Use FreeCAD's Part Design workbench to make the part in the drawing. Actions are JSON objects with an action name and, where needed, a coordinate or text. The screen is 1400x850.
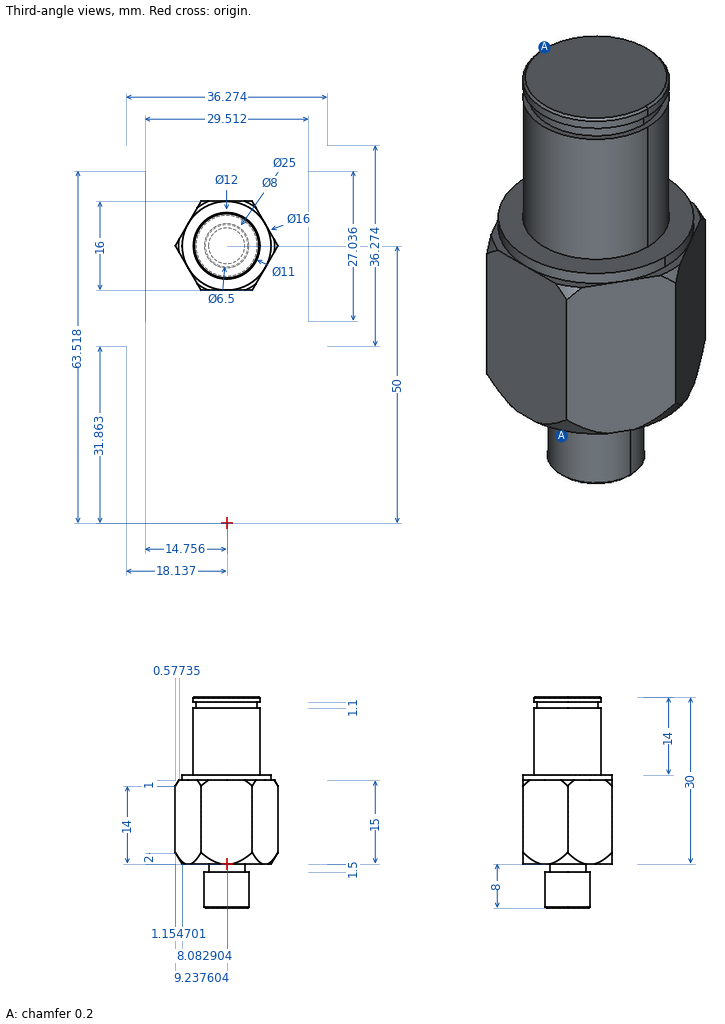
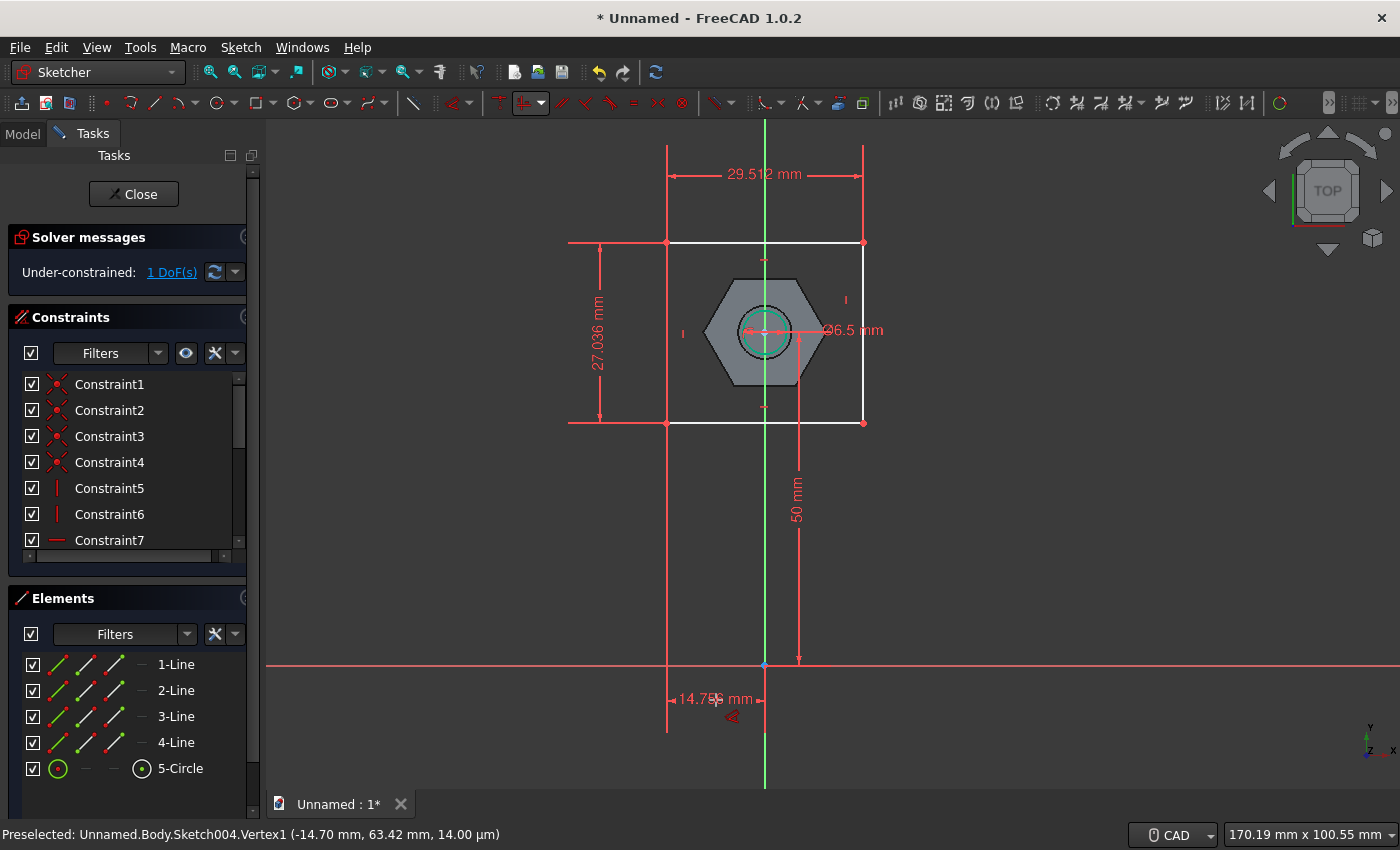
{"action": "left_click", "coordinate": [667, 243]}
{"action": "left_click", "coordinate": [633, 454]}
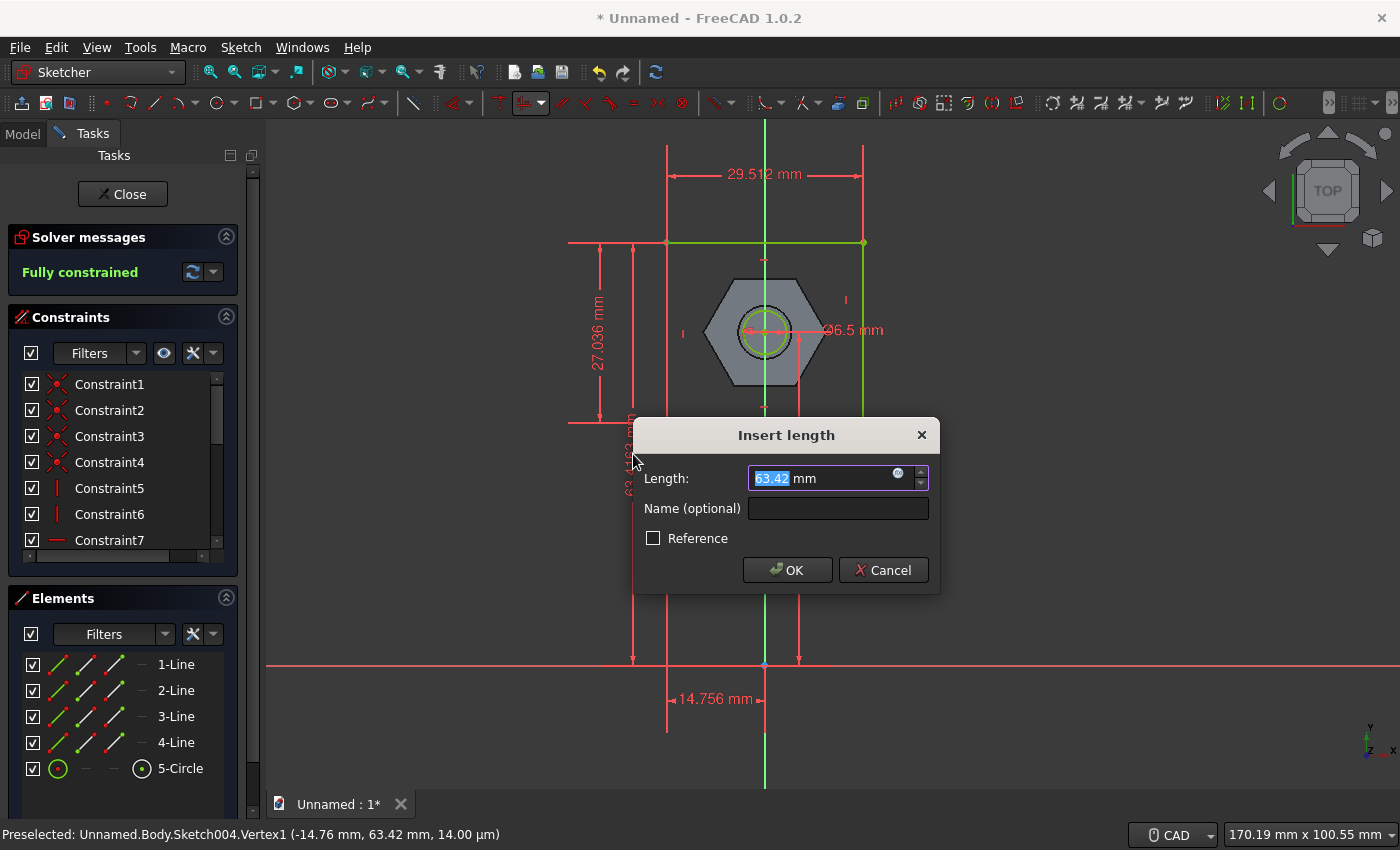
{"action": "type", "text": "63.518"}
{"action": "key", "text": "Return"}
{"action": "key", "text": "Escape"}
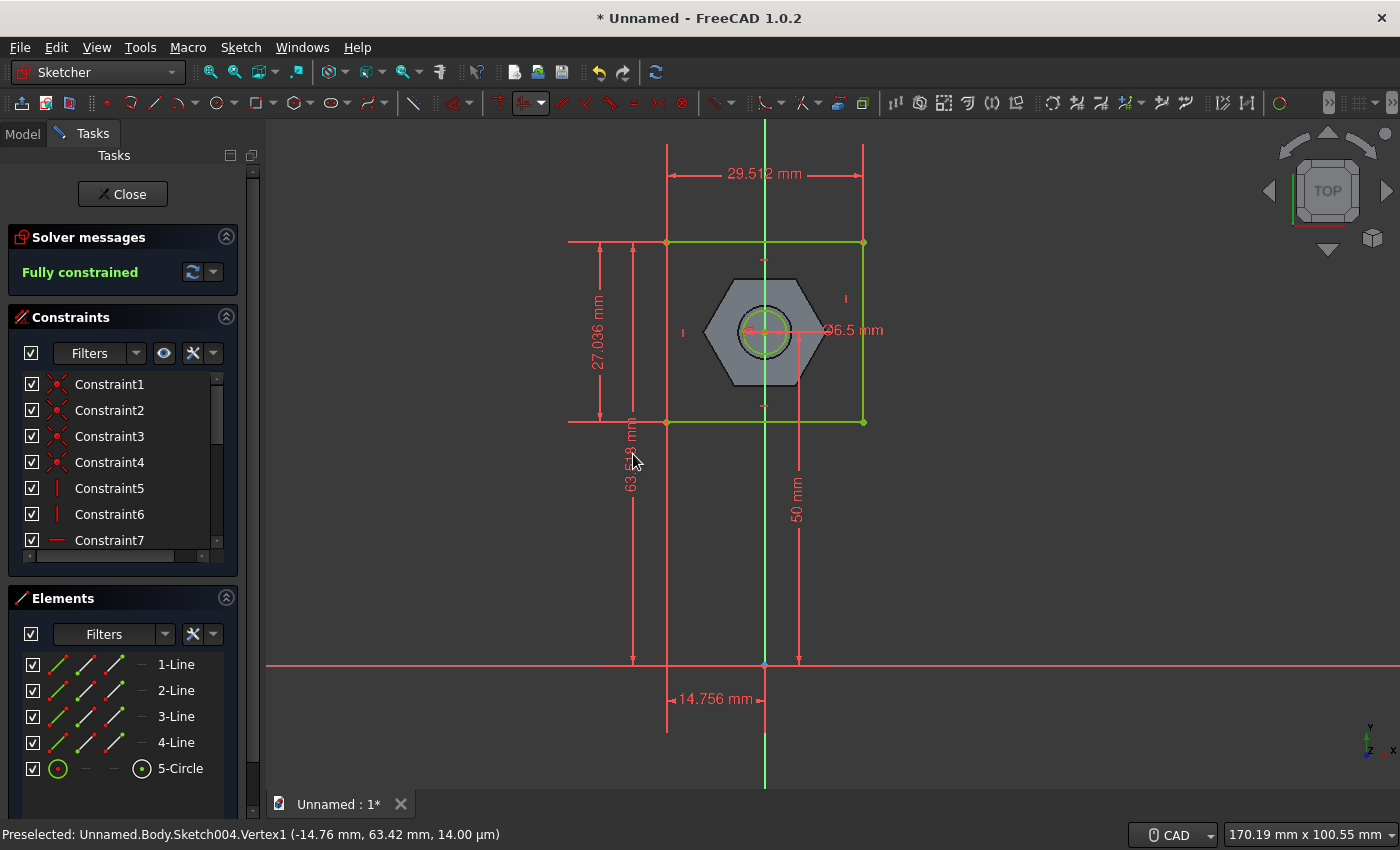
{"action": "left_click", "coordinate": [123, 194]}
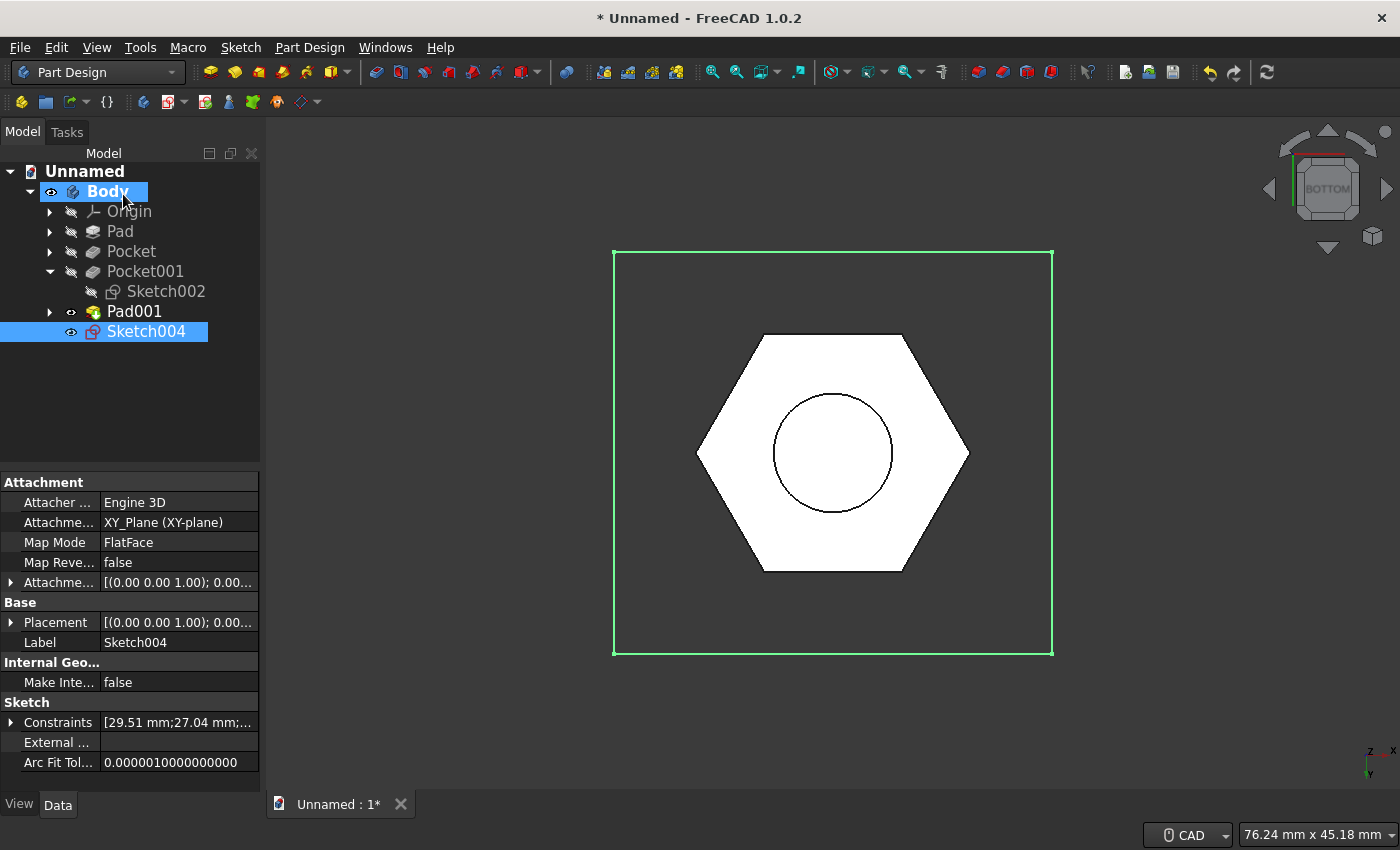
{"action": "left_click", "coordinate": [378, 72]}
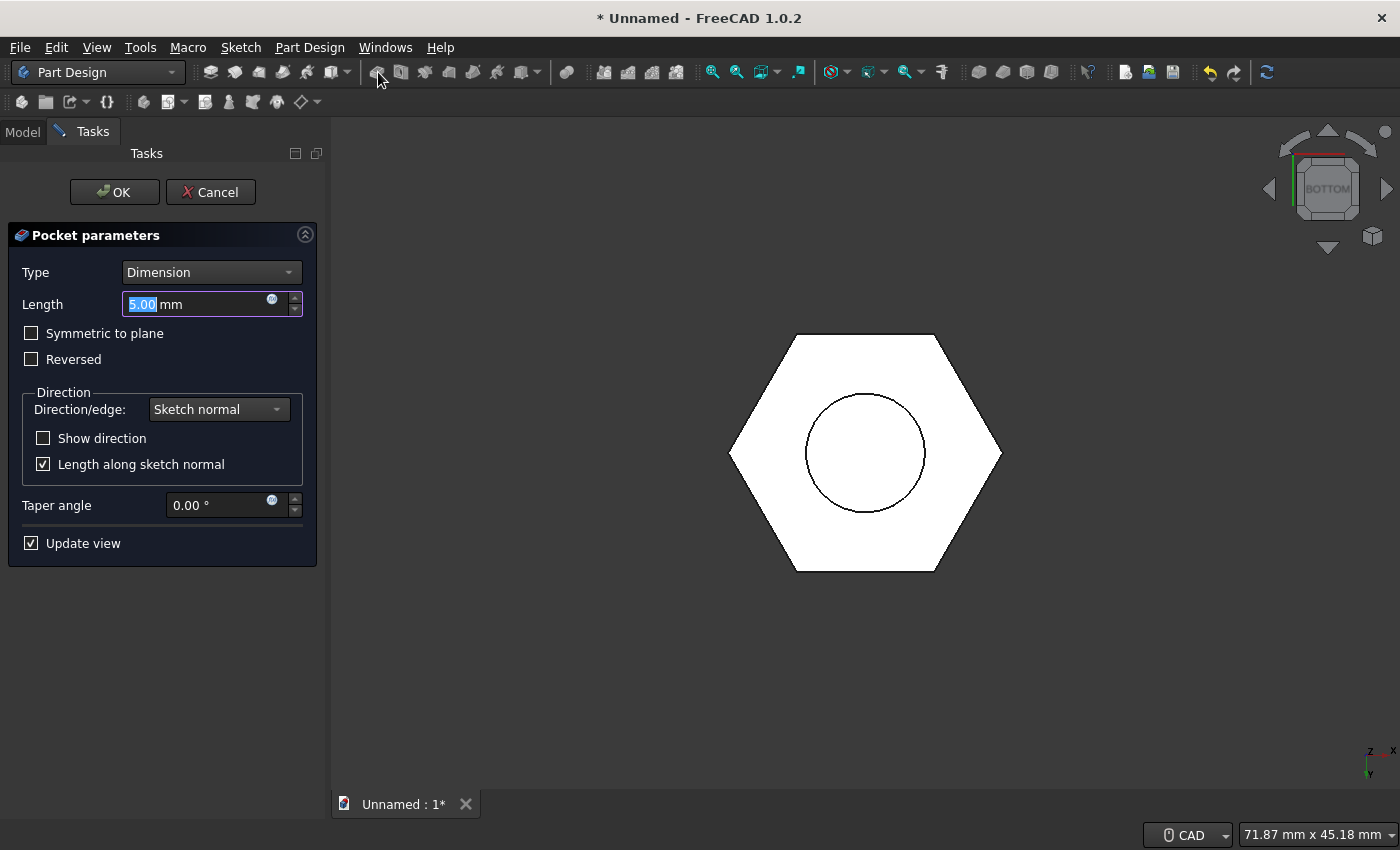
{"action": "type", "text": "1.5"}
{"action": "key", "text": "Tab"}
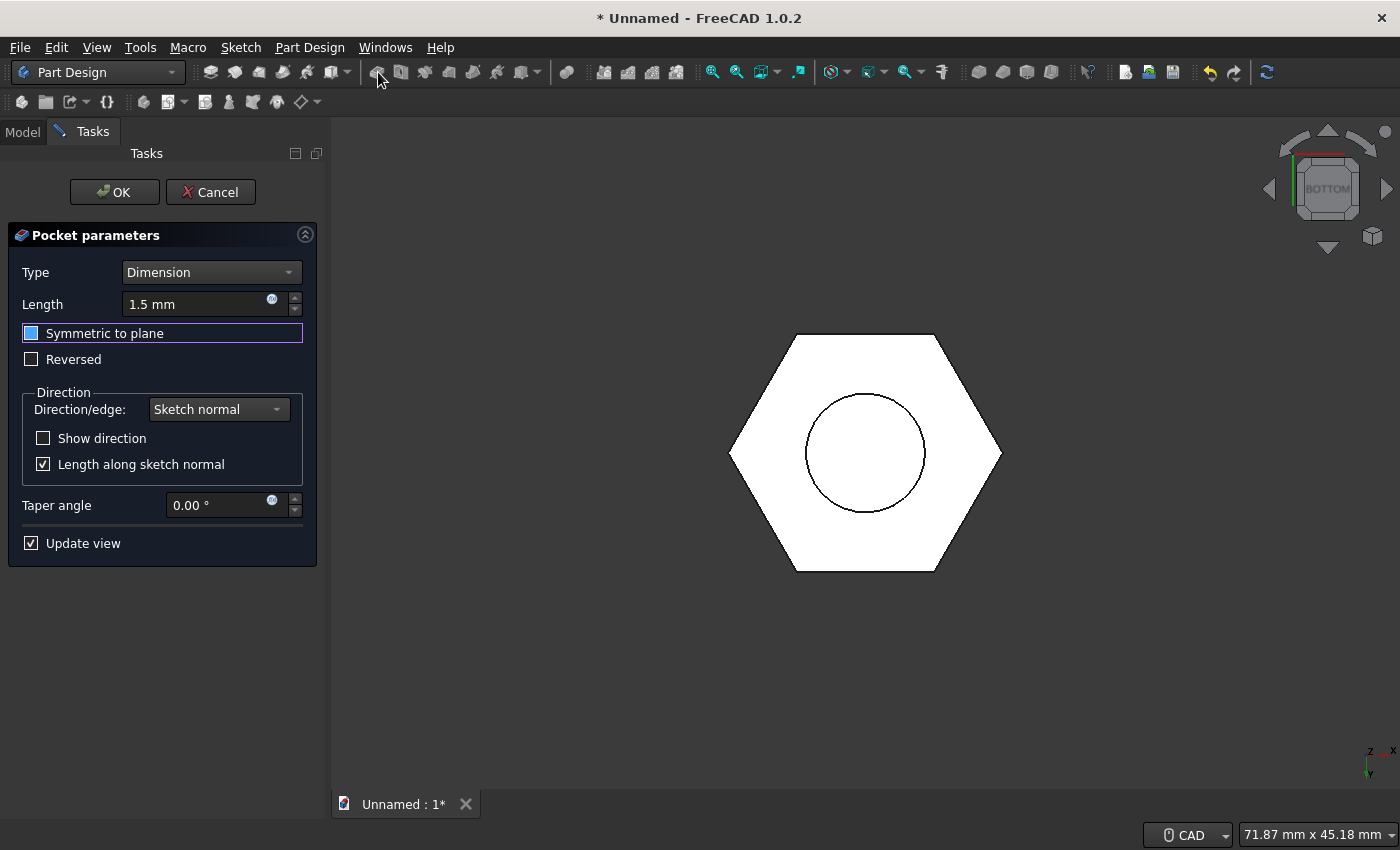
{"action": "left_click", "coordinate": [115, 192]}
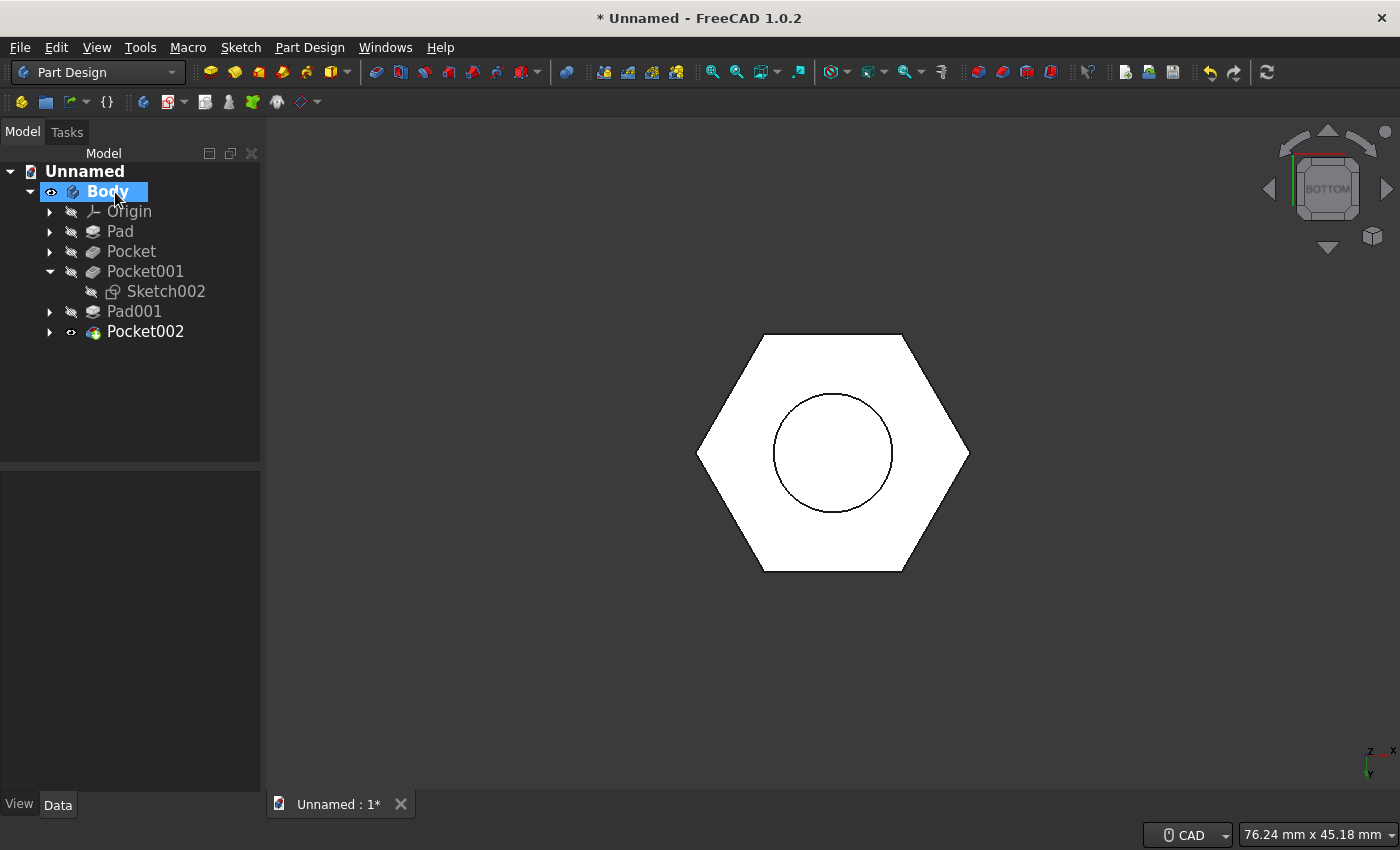
{"action": "left_click", "coordinate": [714, 72]}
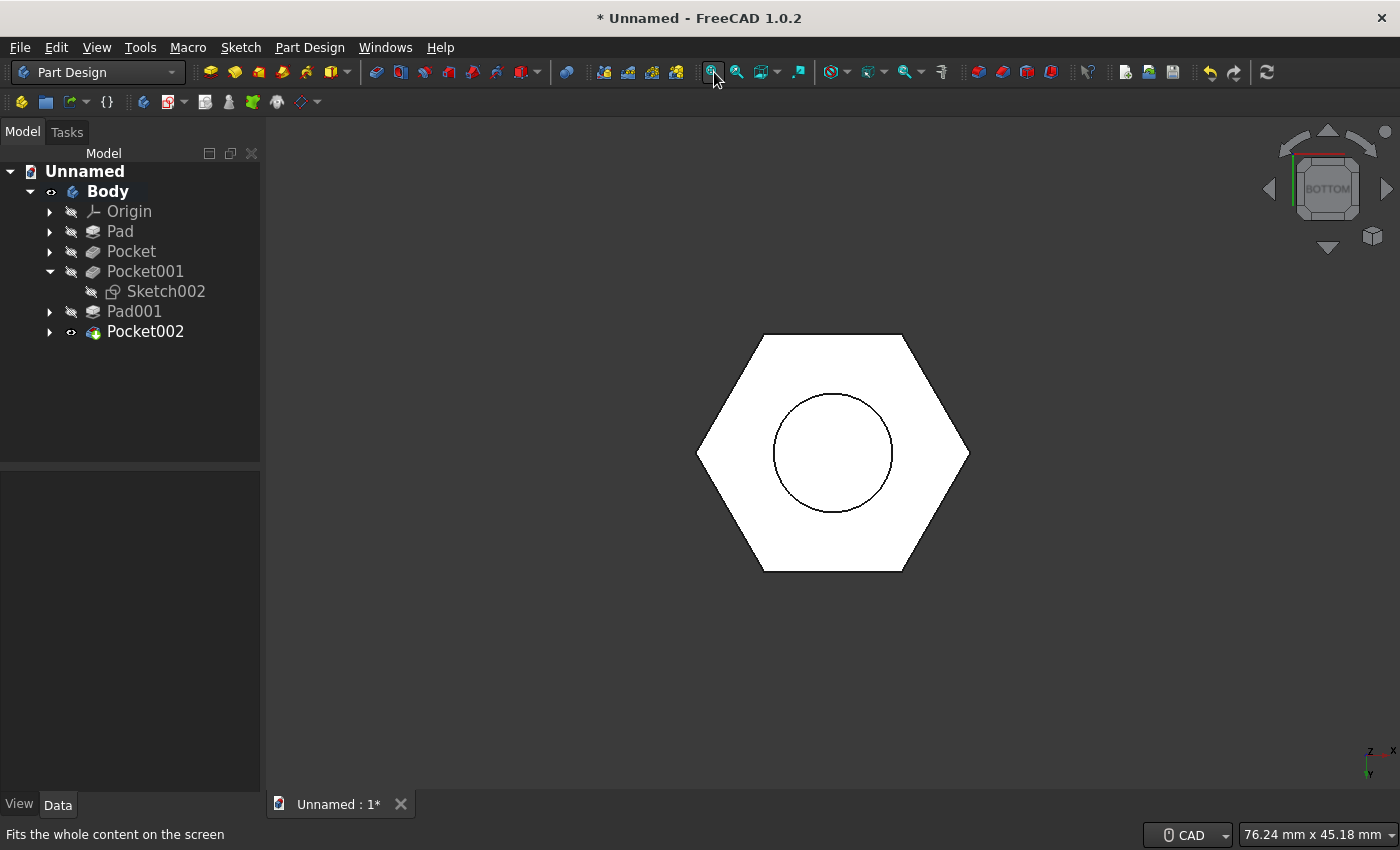
{"action": "key", "text": "0"}